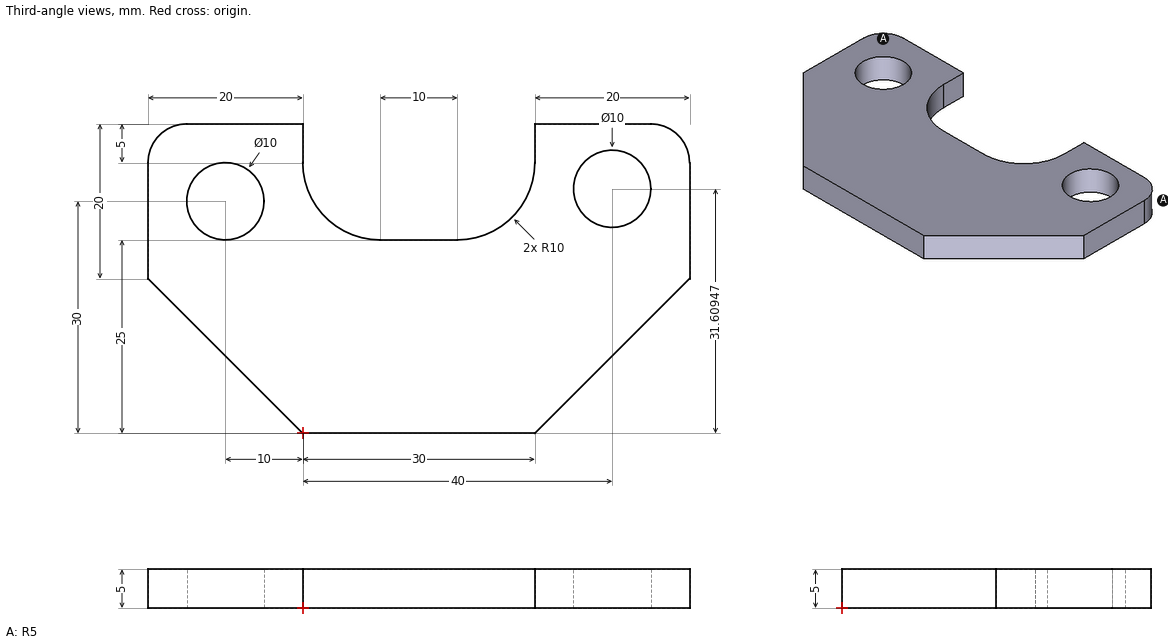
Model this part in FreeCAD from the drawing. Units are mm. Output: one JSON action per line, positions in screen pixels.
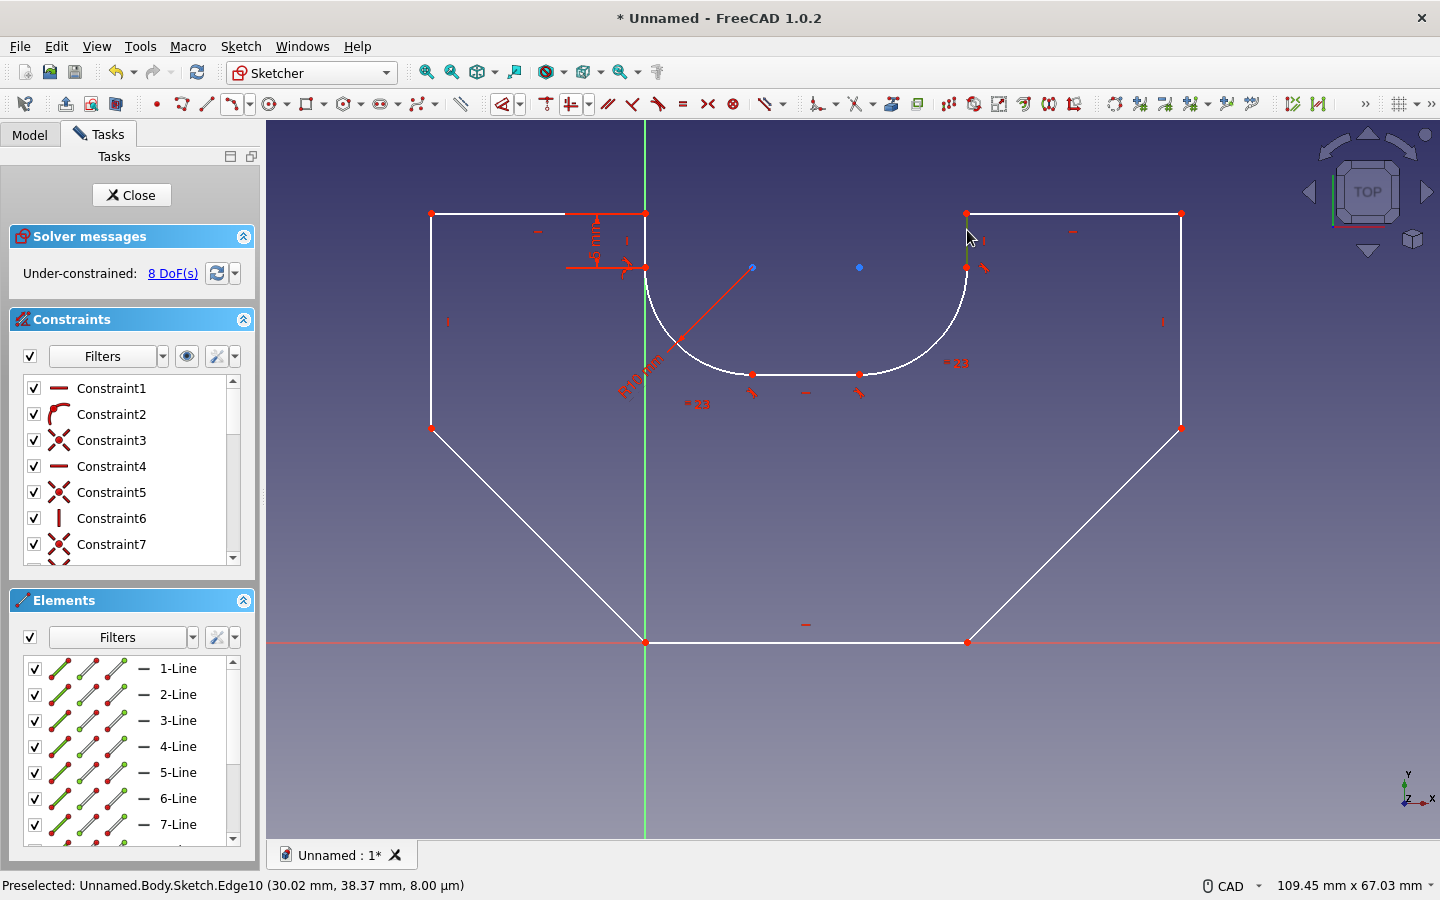
{"action": "key", "text": "i"}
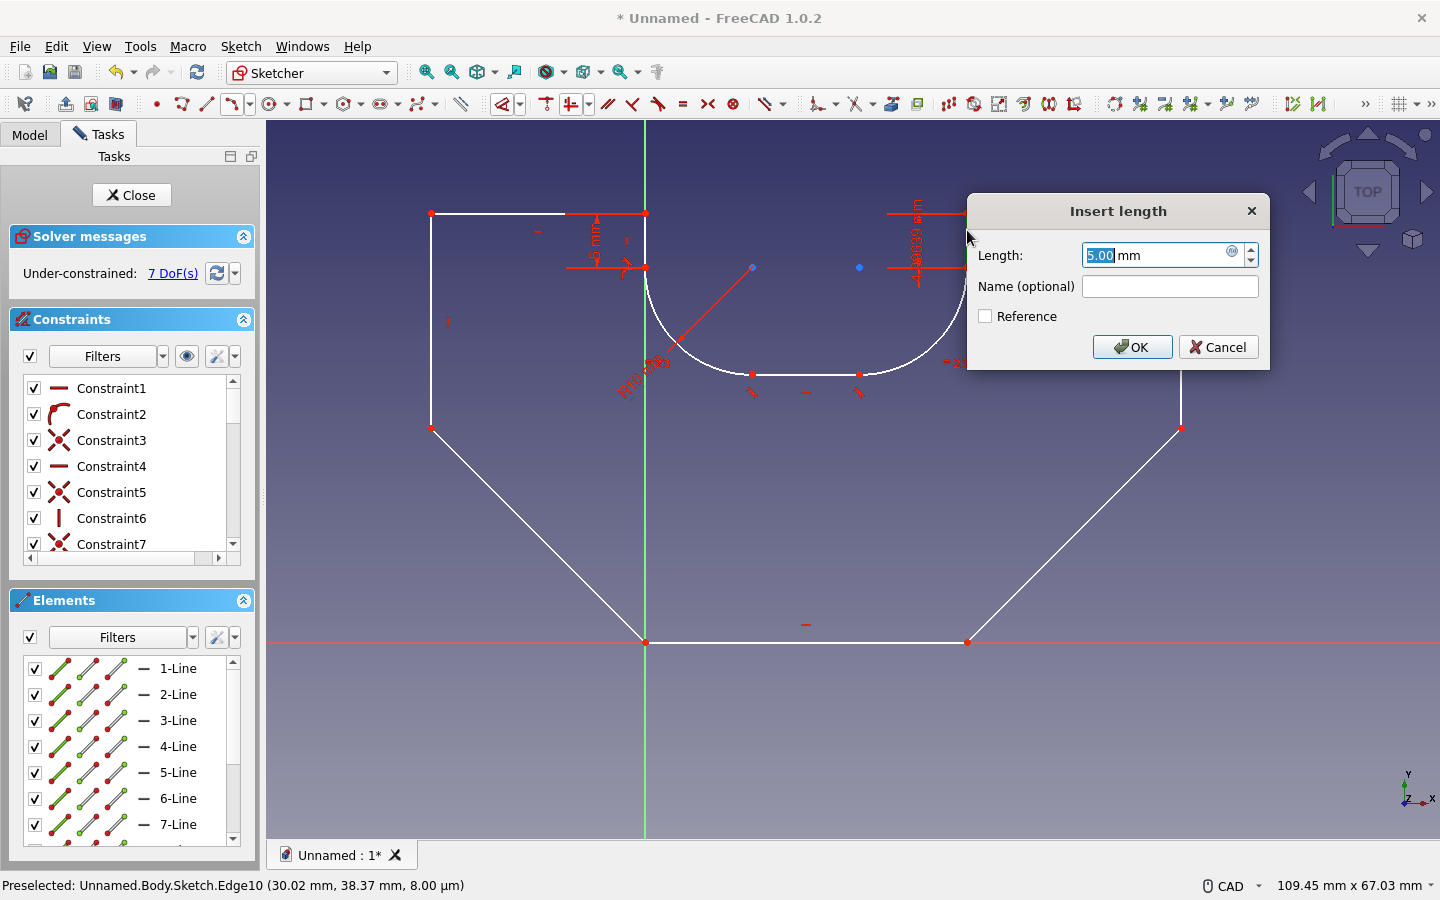
{"action": "type", "text": "5"}
{"action": "key", "text": "Return"}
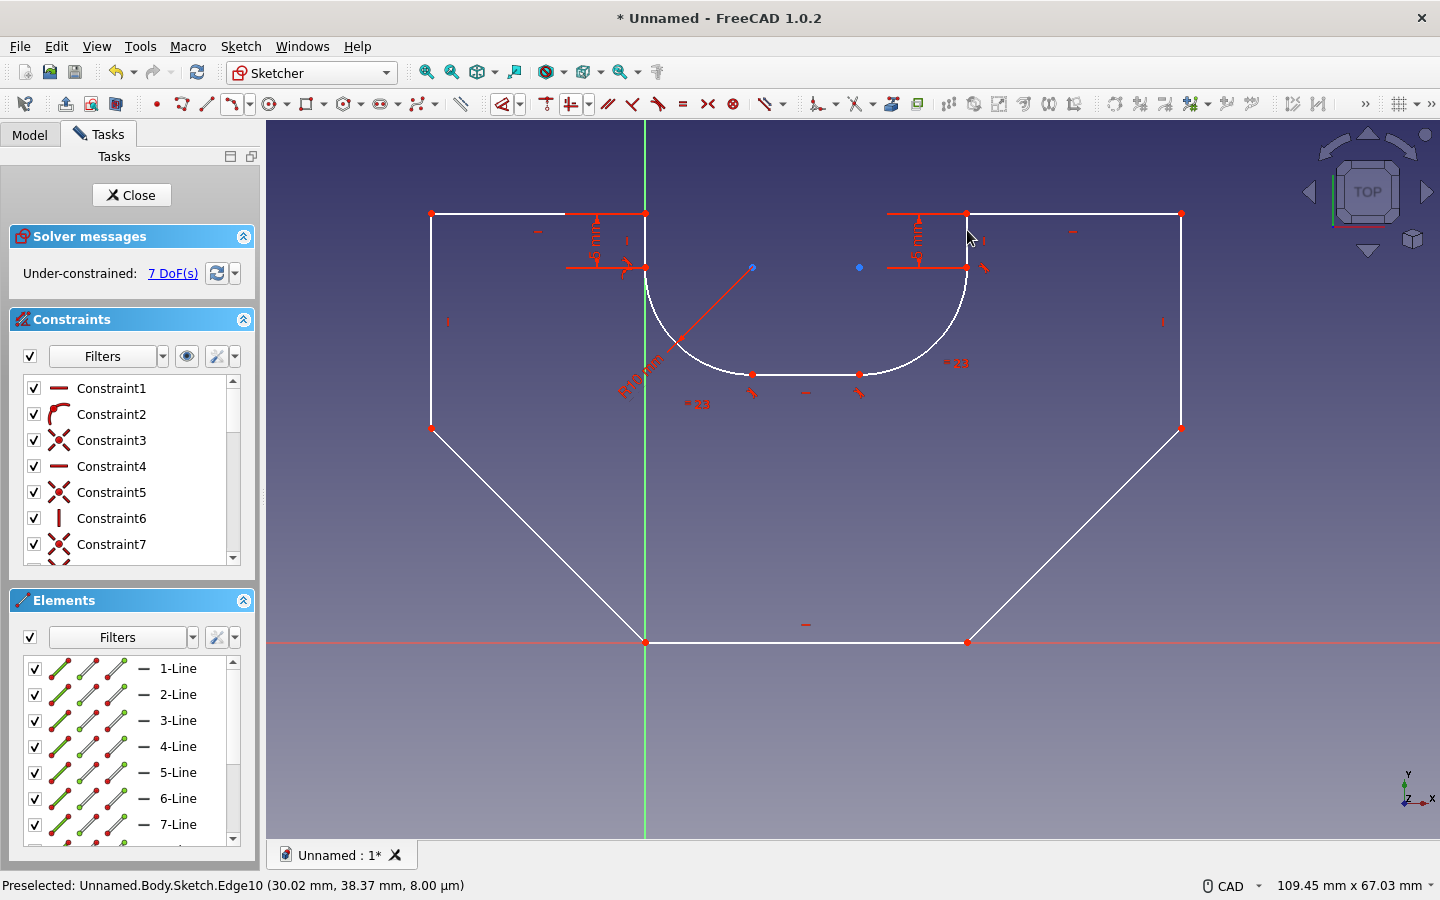
{"action": "left_click", "coordinate": [828, 375]}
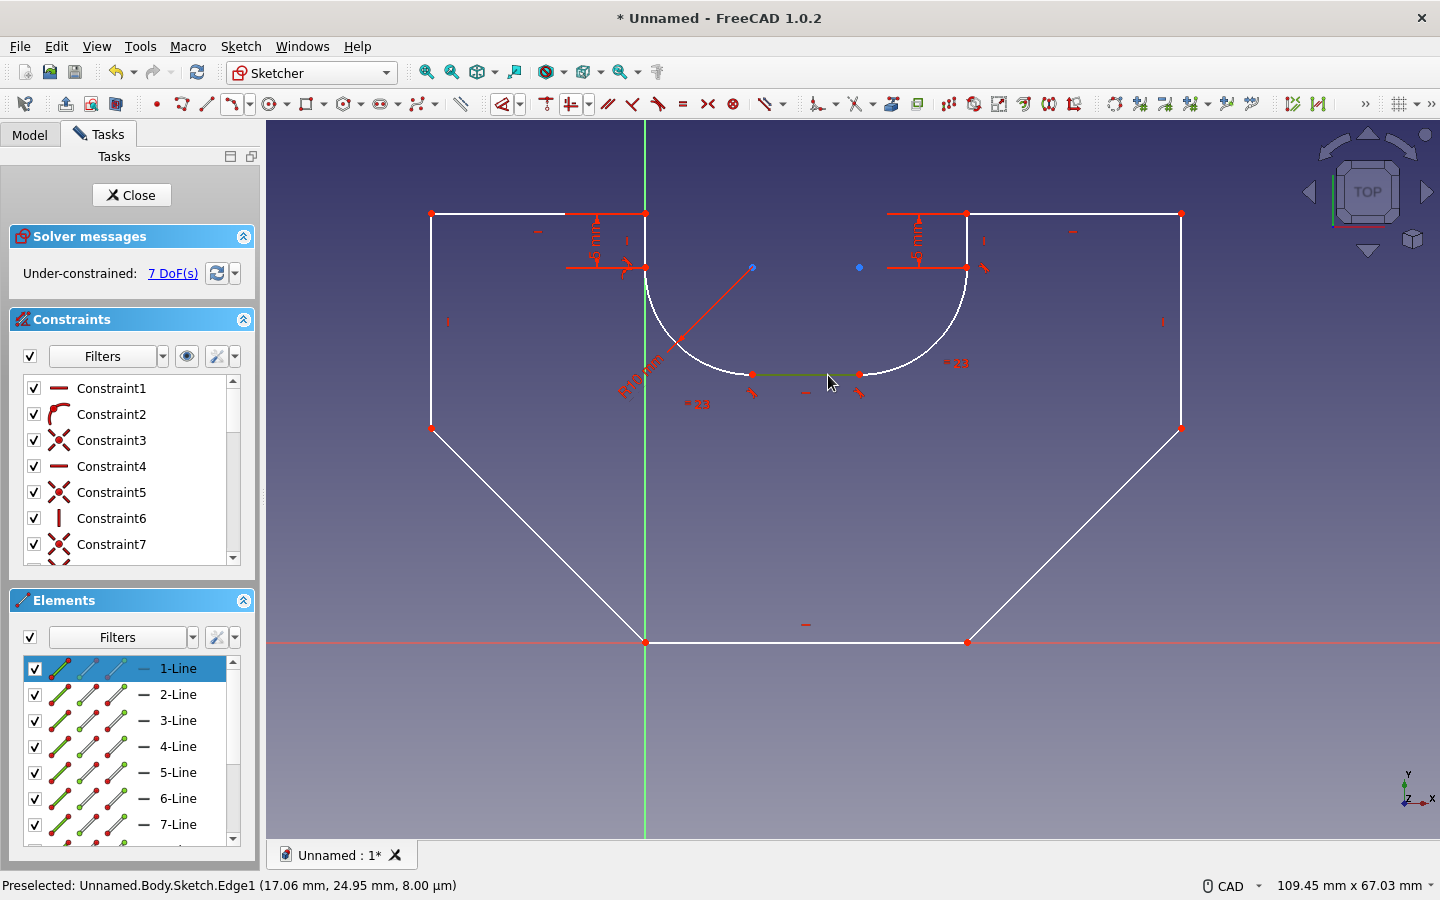
{"action": "key", "text": "l"}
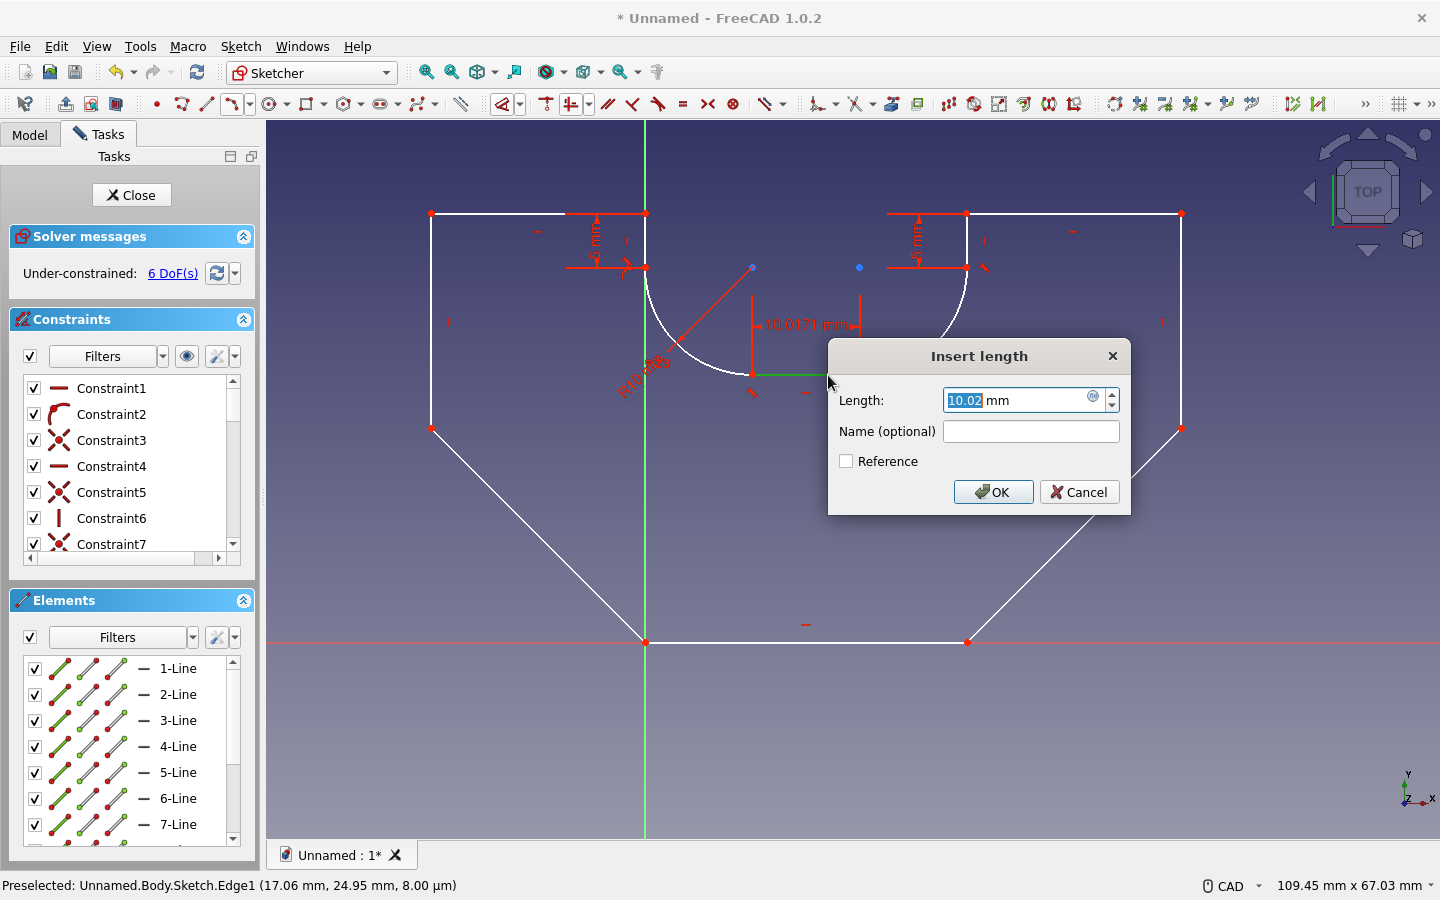
{"action": "type", "text": "10"}
{"action": "key", "text": "Return"}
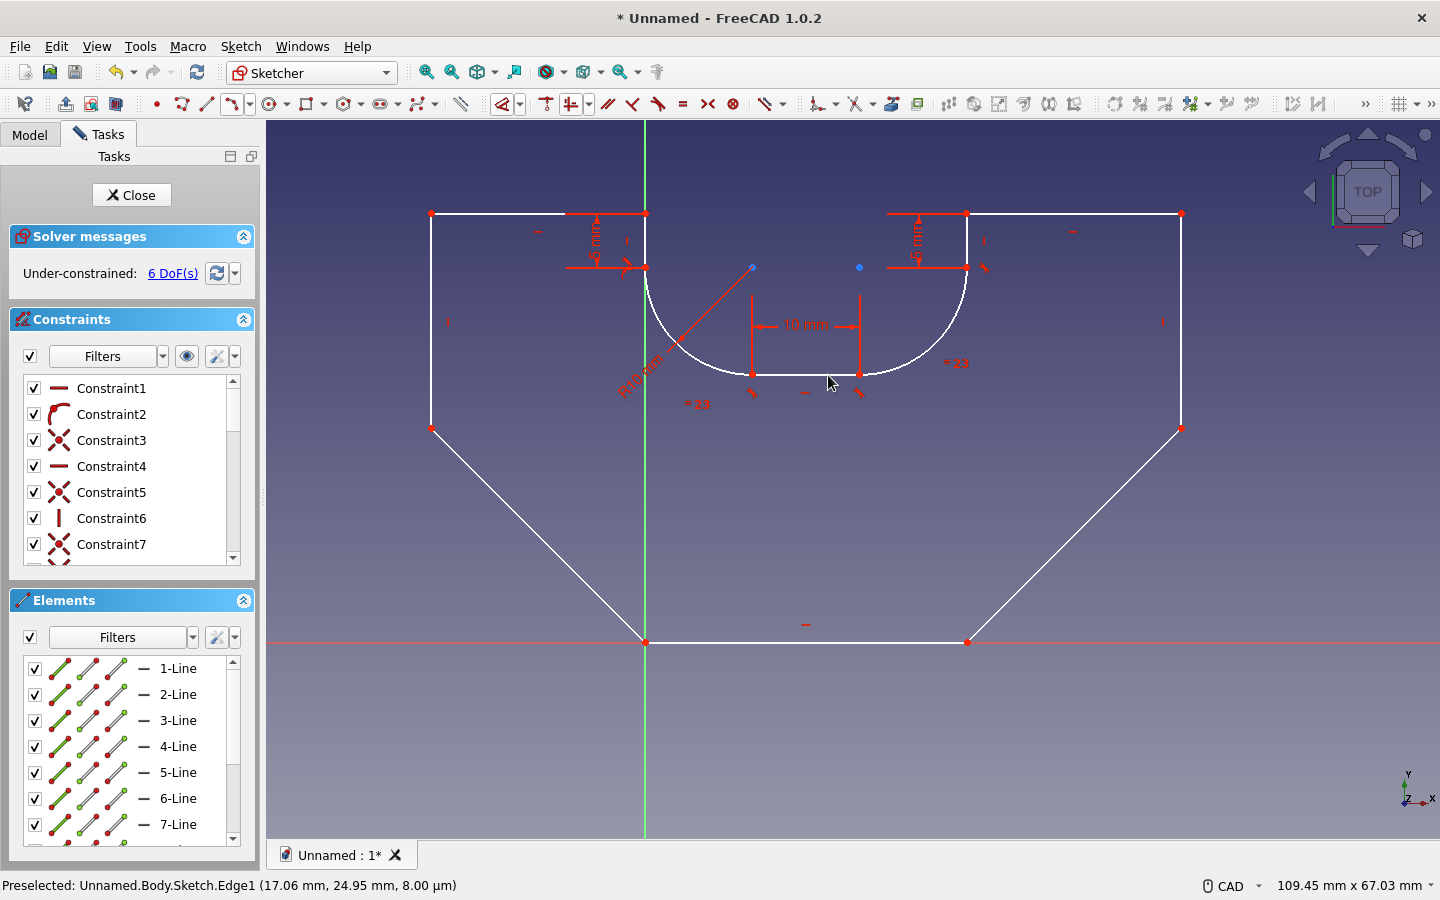
{"action": "left_click", "coordinate": [581, 214]}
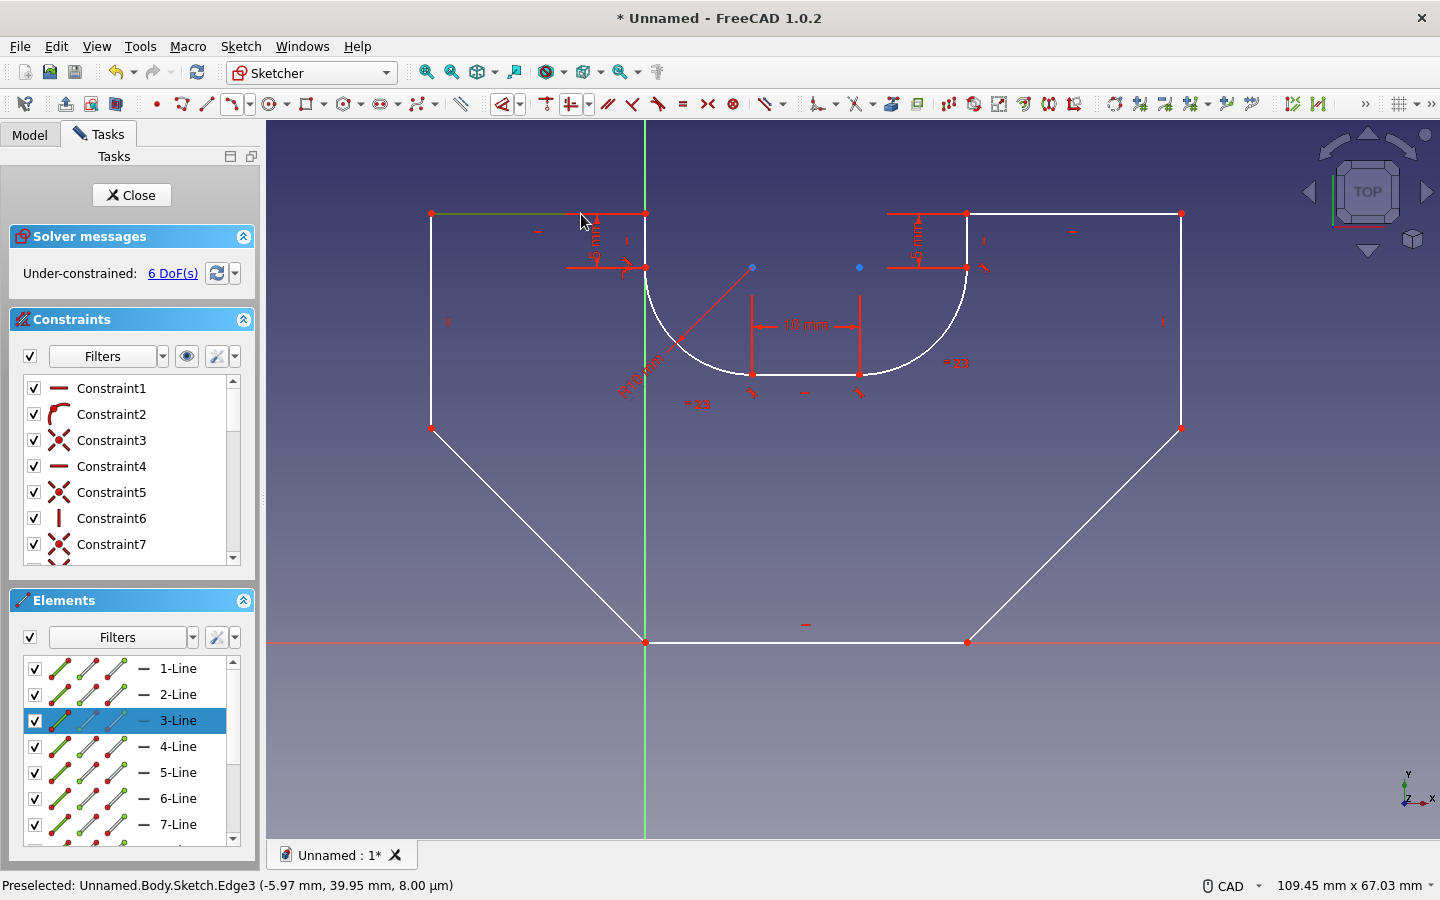
{"action": "left_click", "coordinate": [520, 104]}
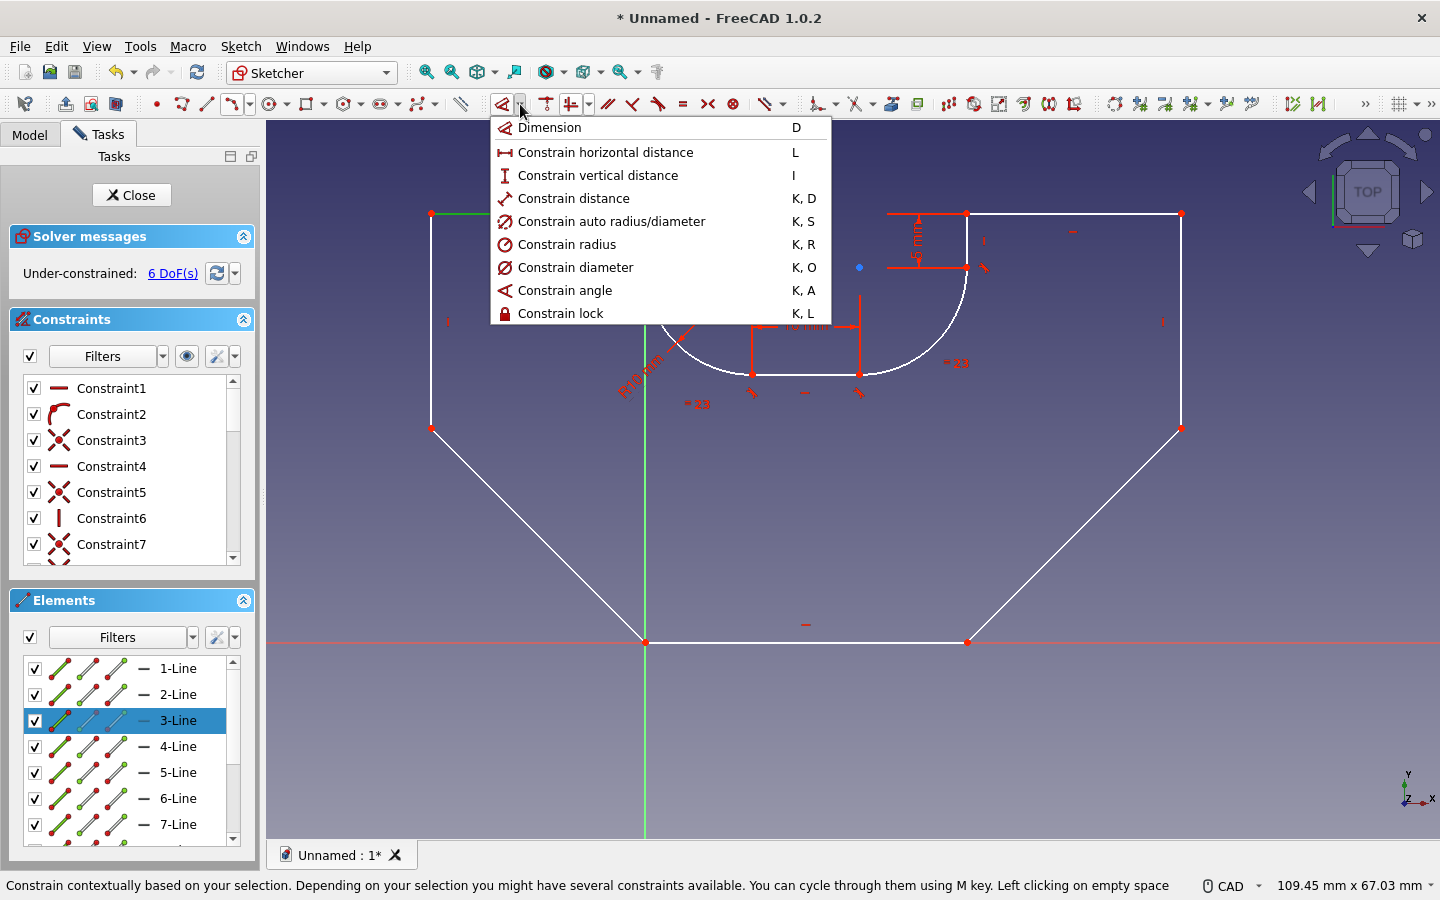
{"action": "left_click", "coordinate": [661, 152]}